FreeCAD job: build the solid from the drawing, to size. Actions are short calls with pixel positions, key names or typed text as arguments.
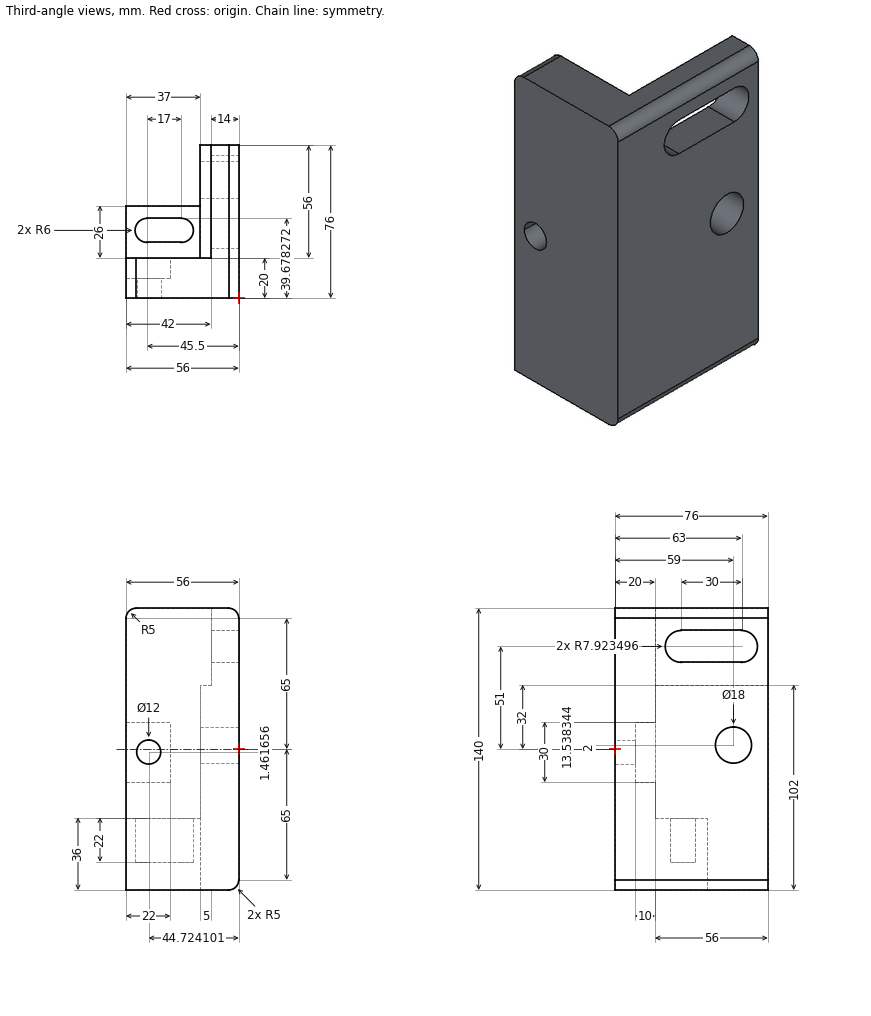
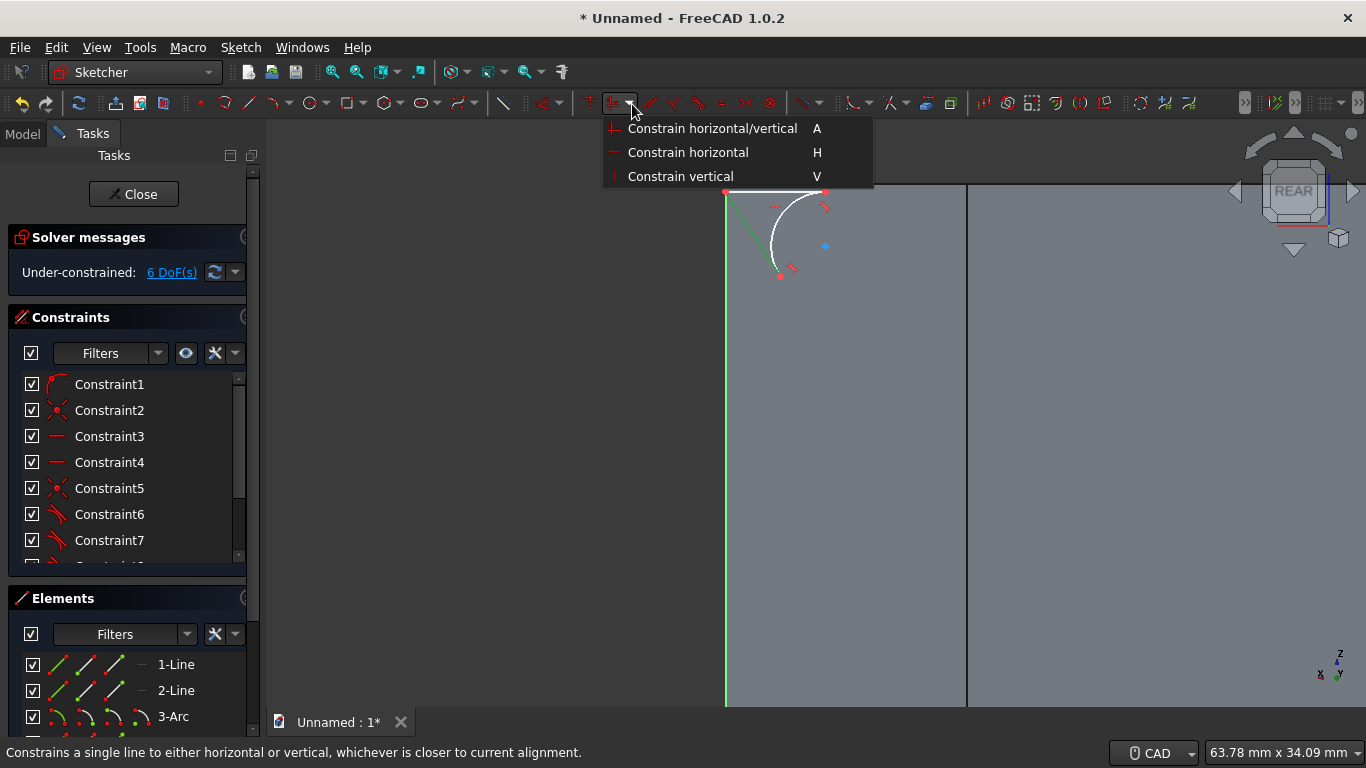
click(738, 176)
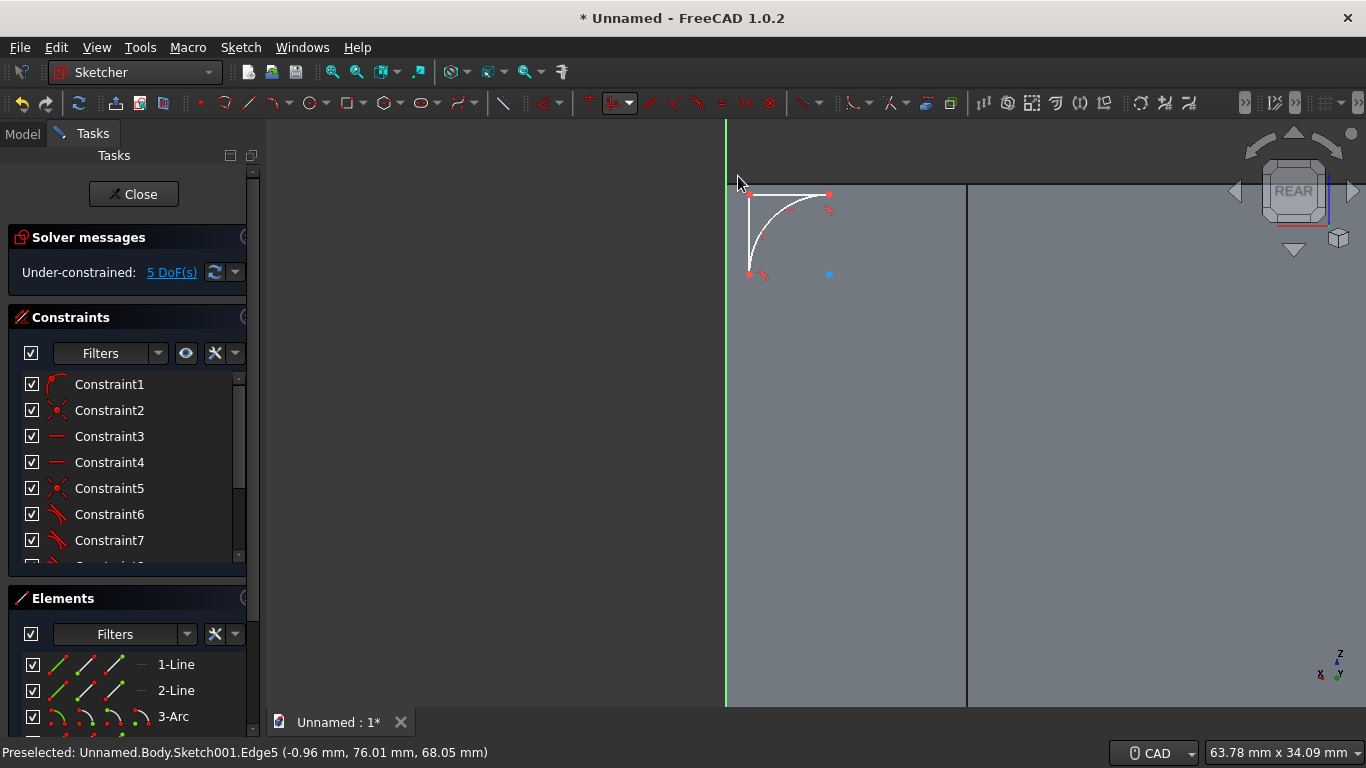
scroll(743, 219, down, 9)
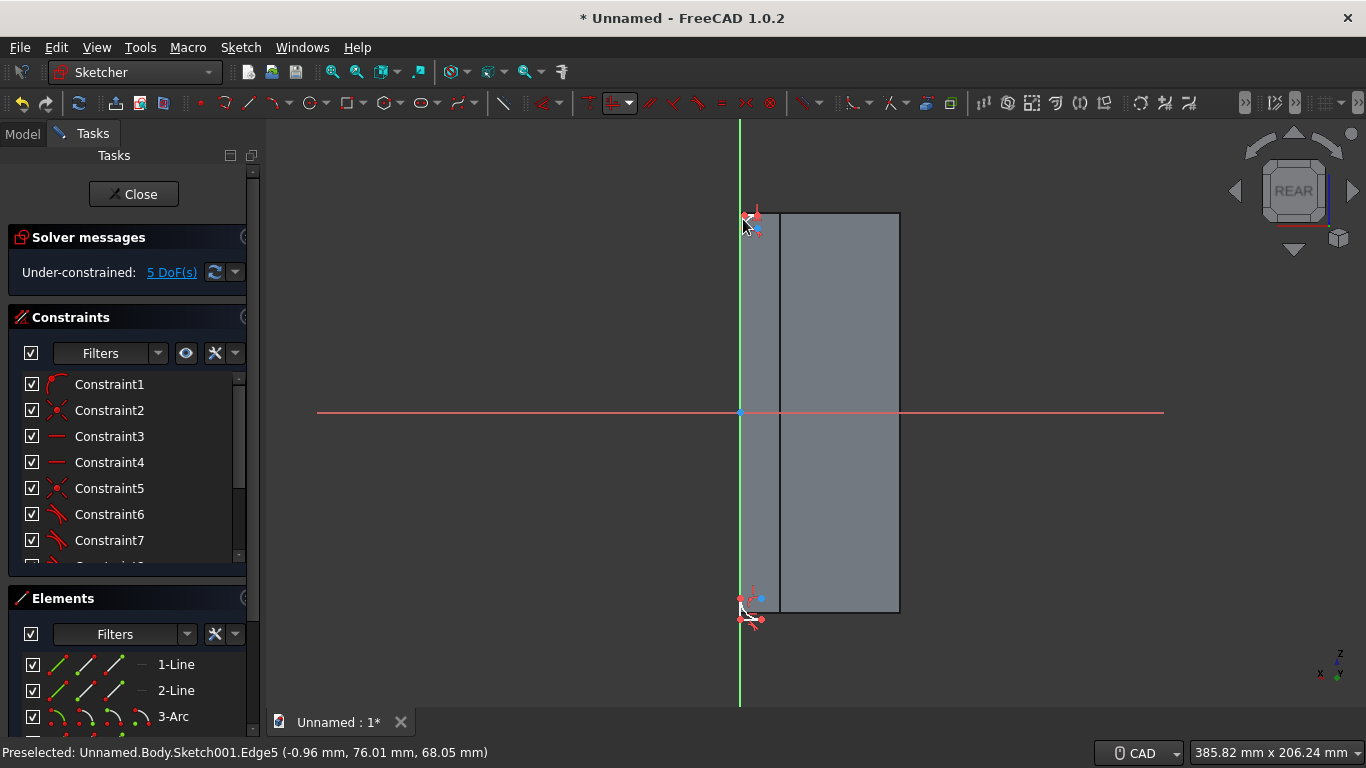
scroll(743, 608, up, 9)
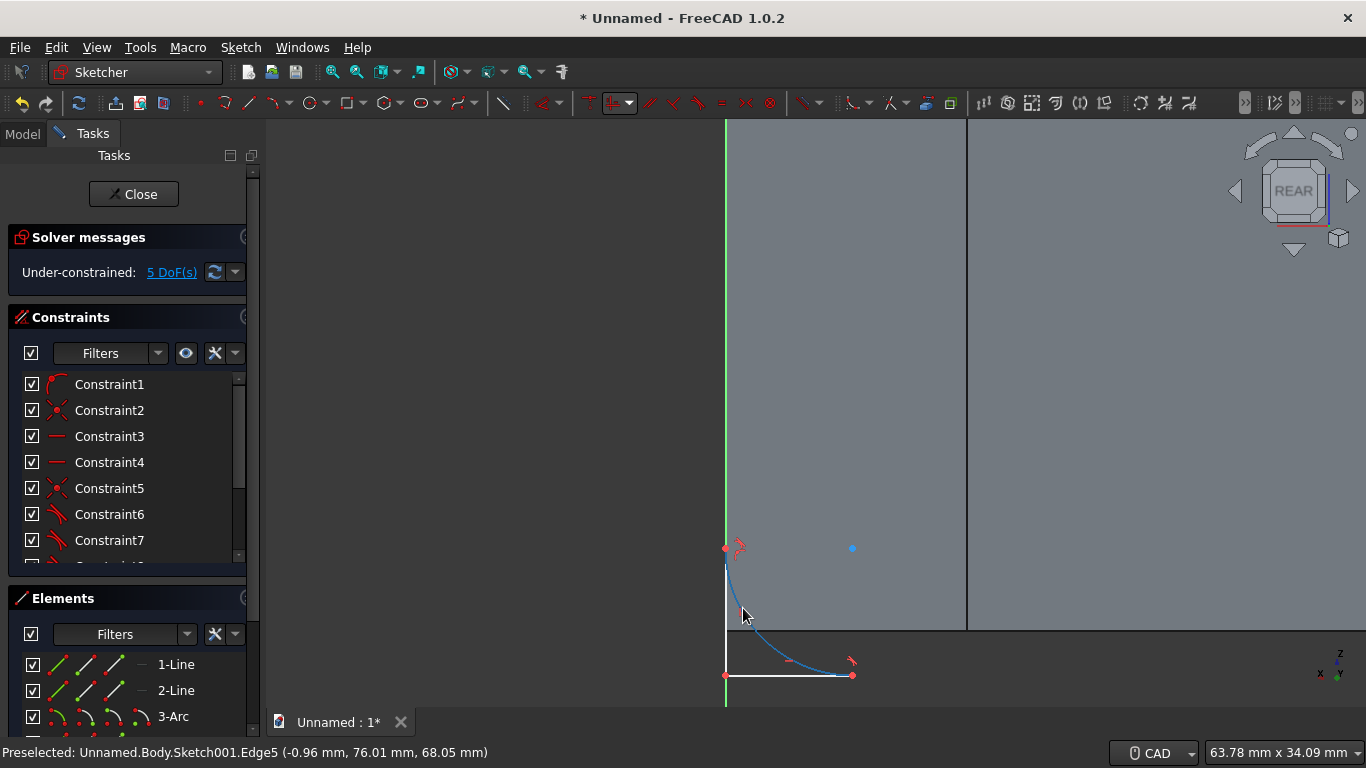
click(763, 638)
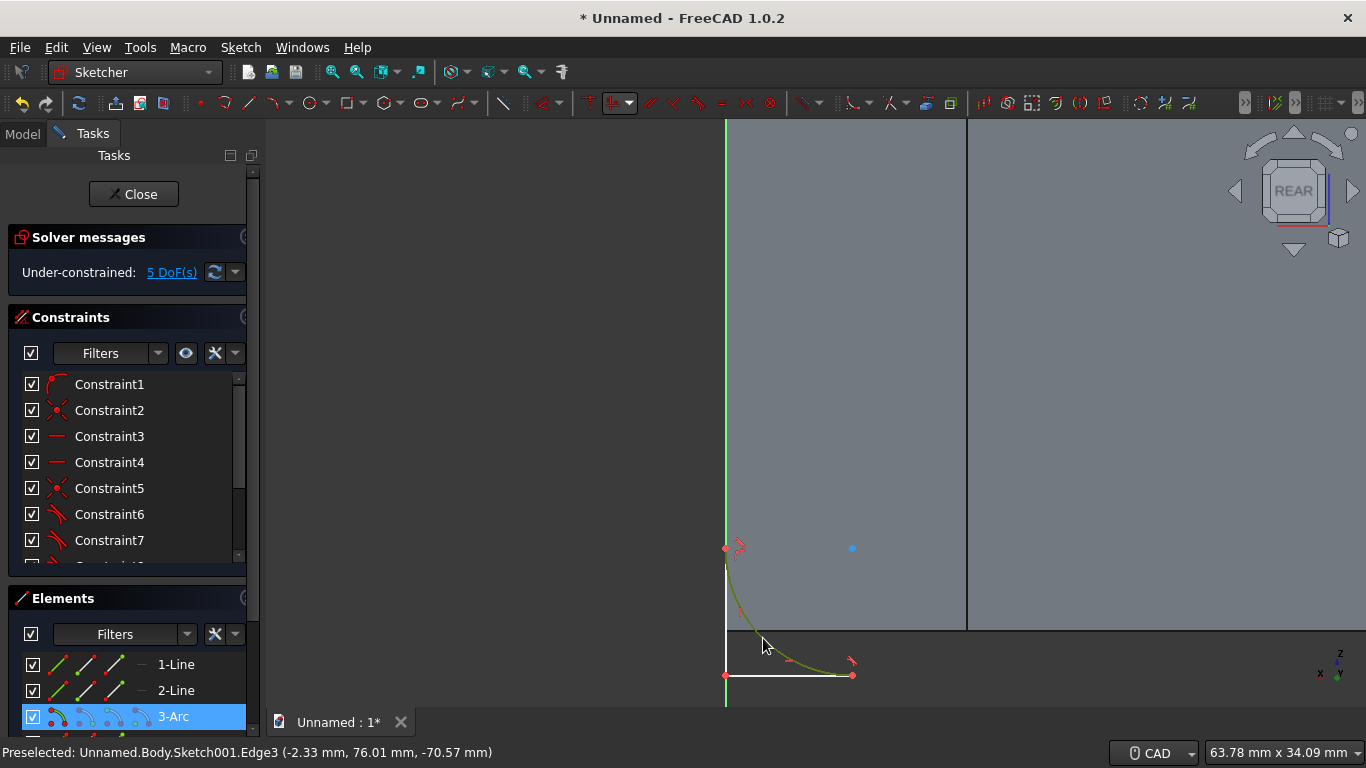
scroll(743, 609, down, 9)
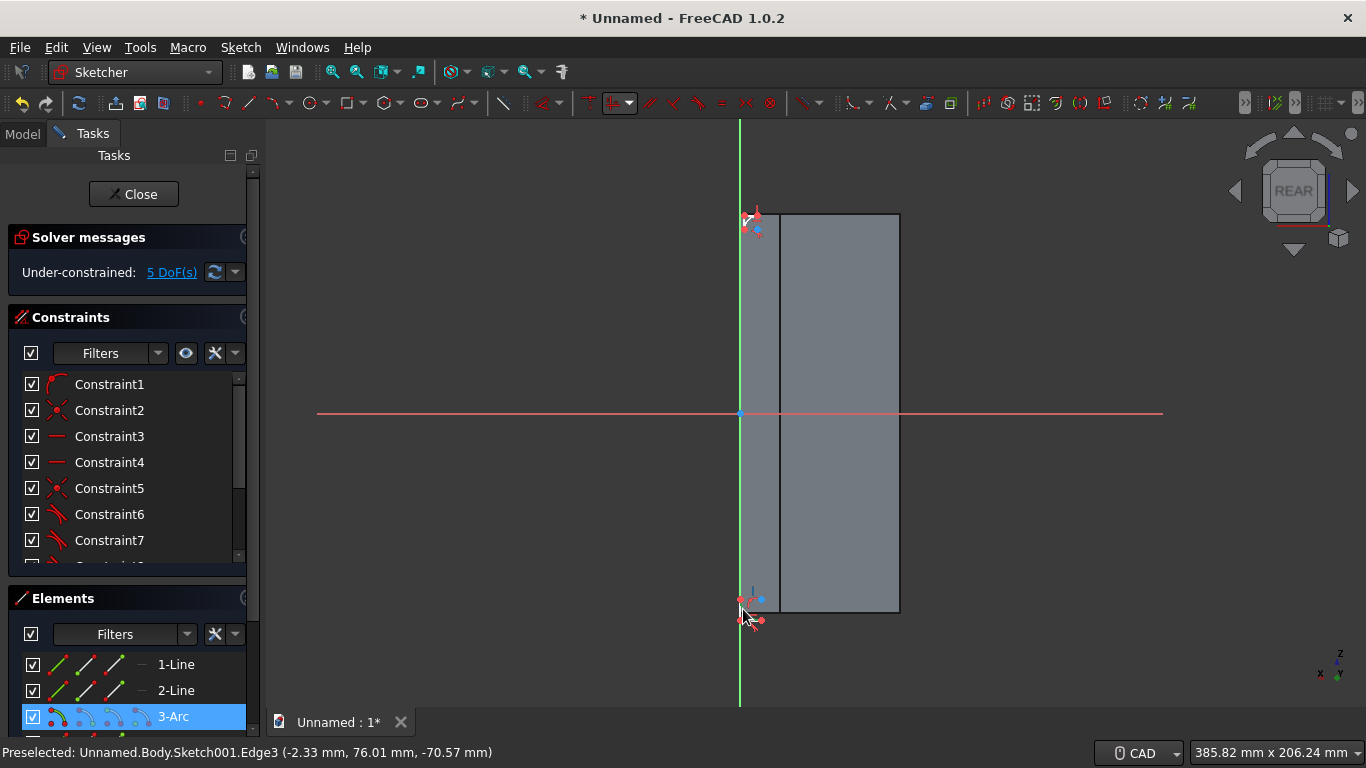
scroll(748, 220, up, 7)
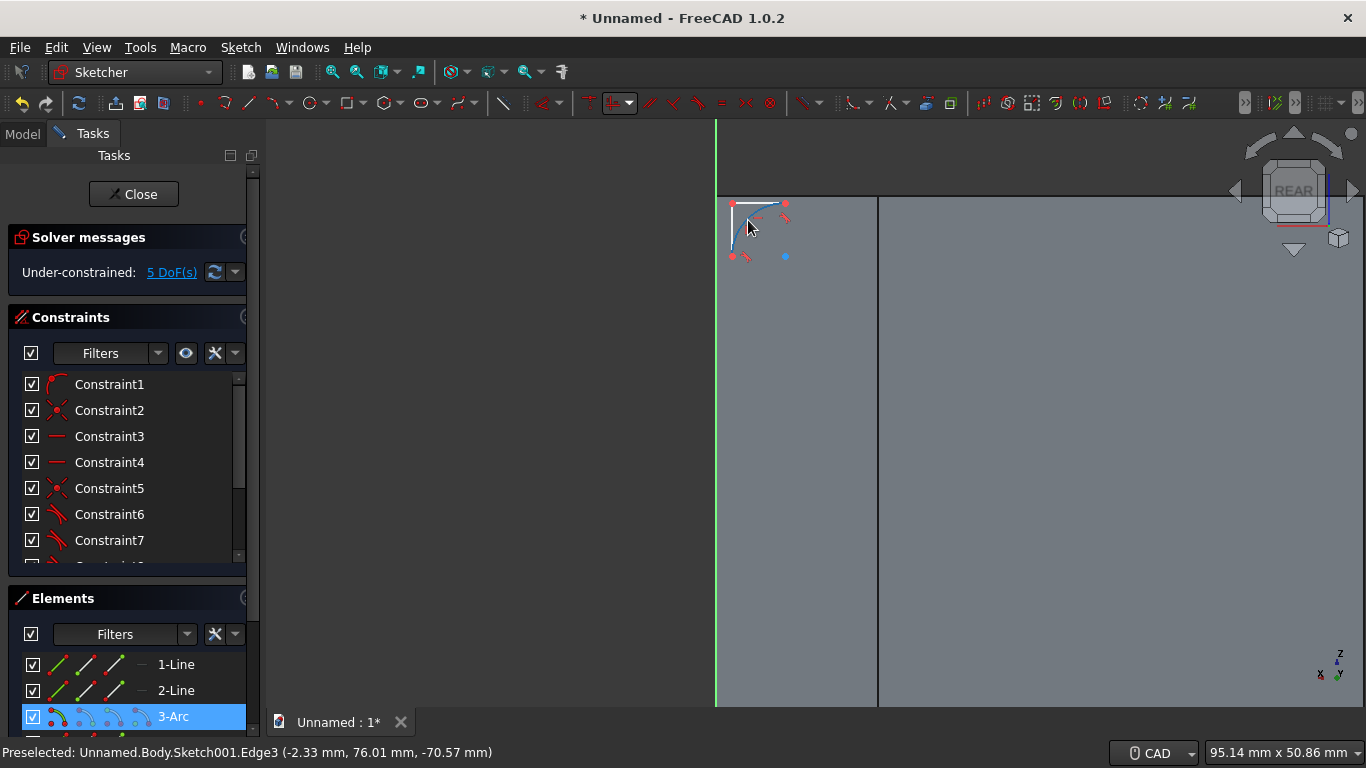
click(748, 219)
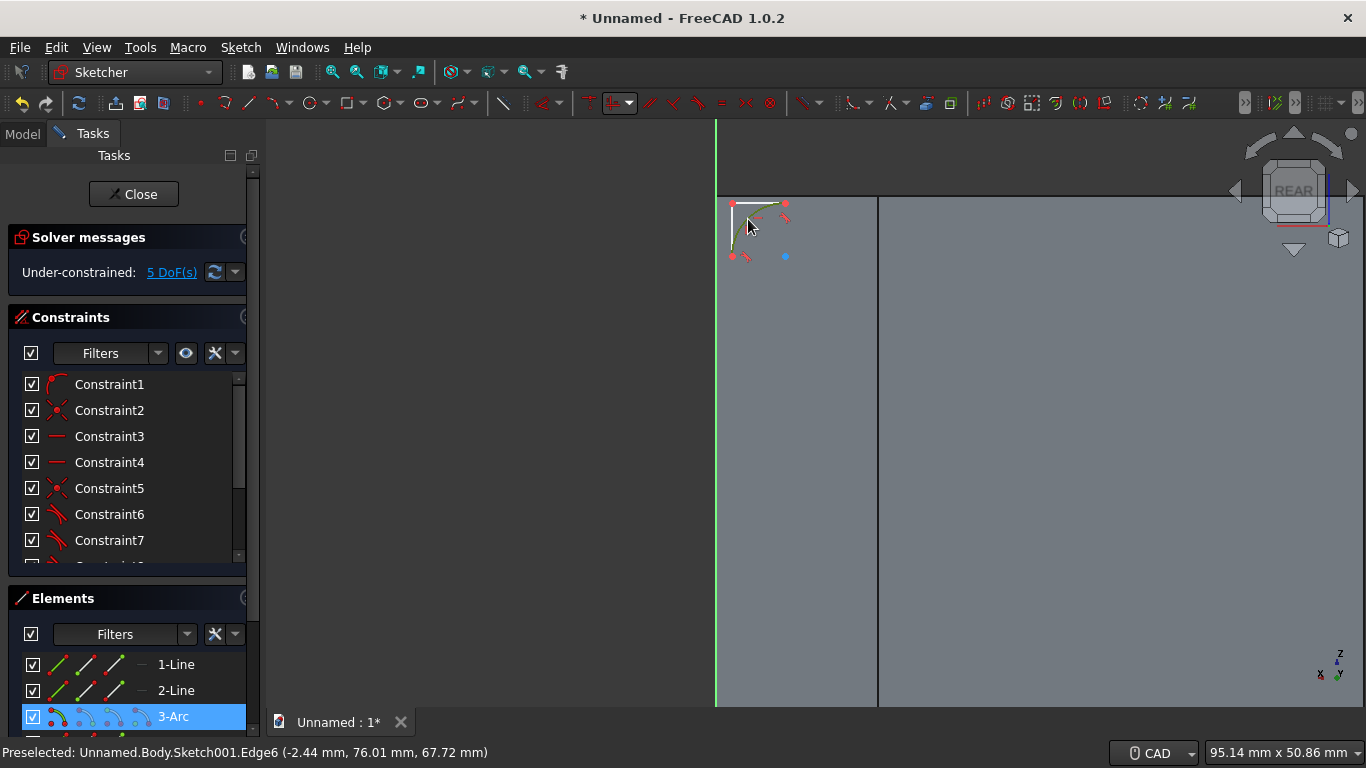
click(722, 104)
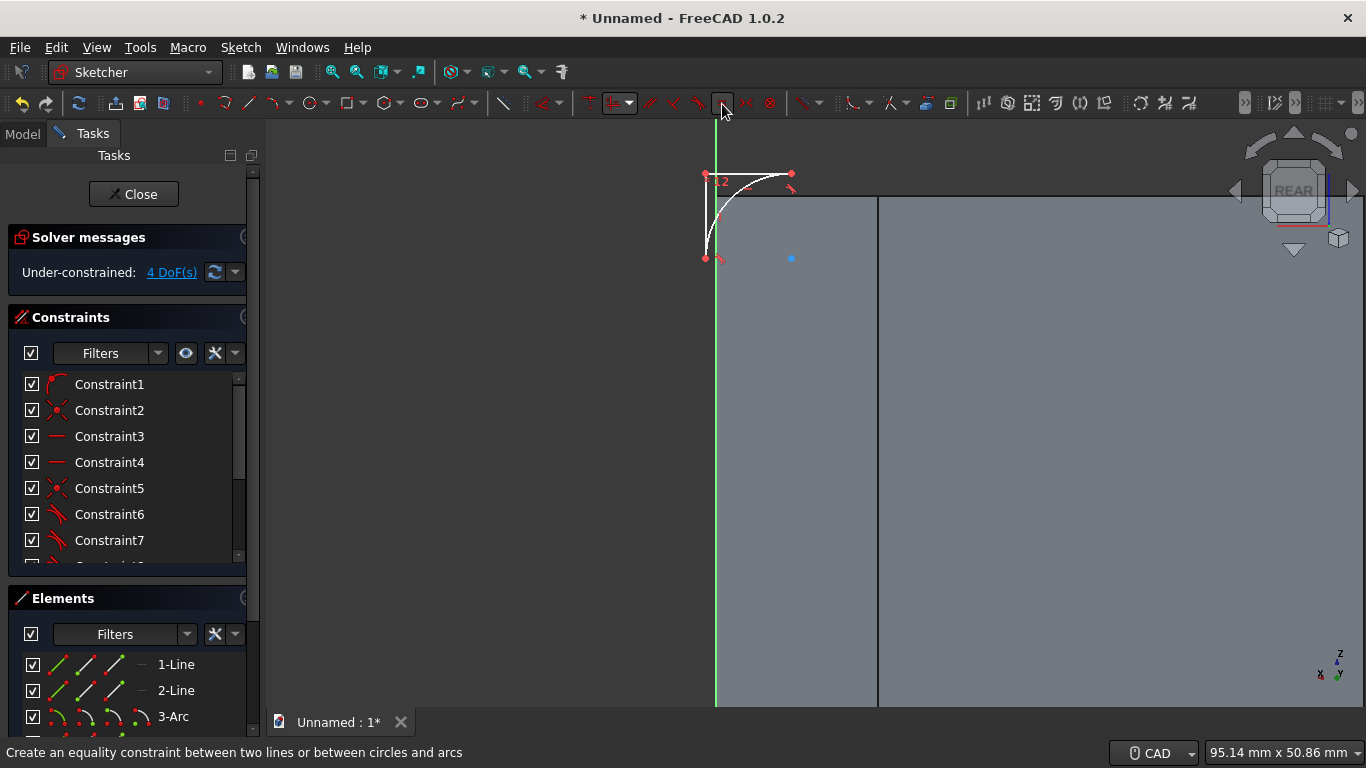
scroll(748, 219, down, 7)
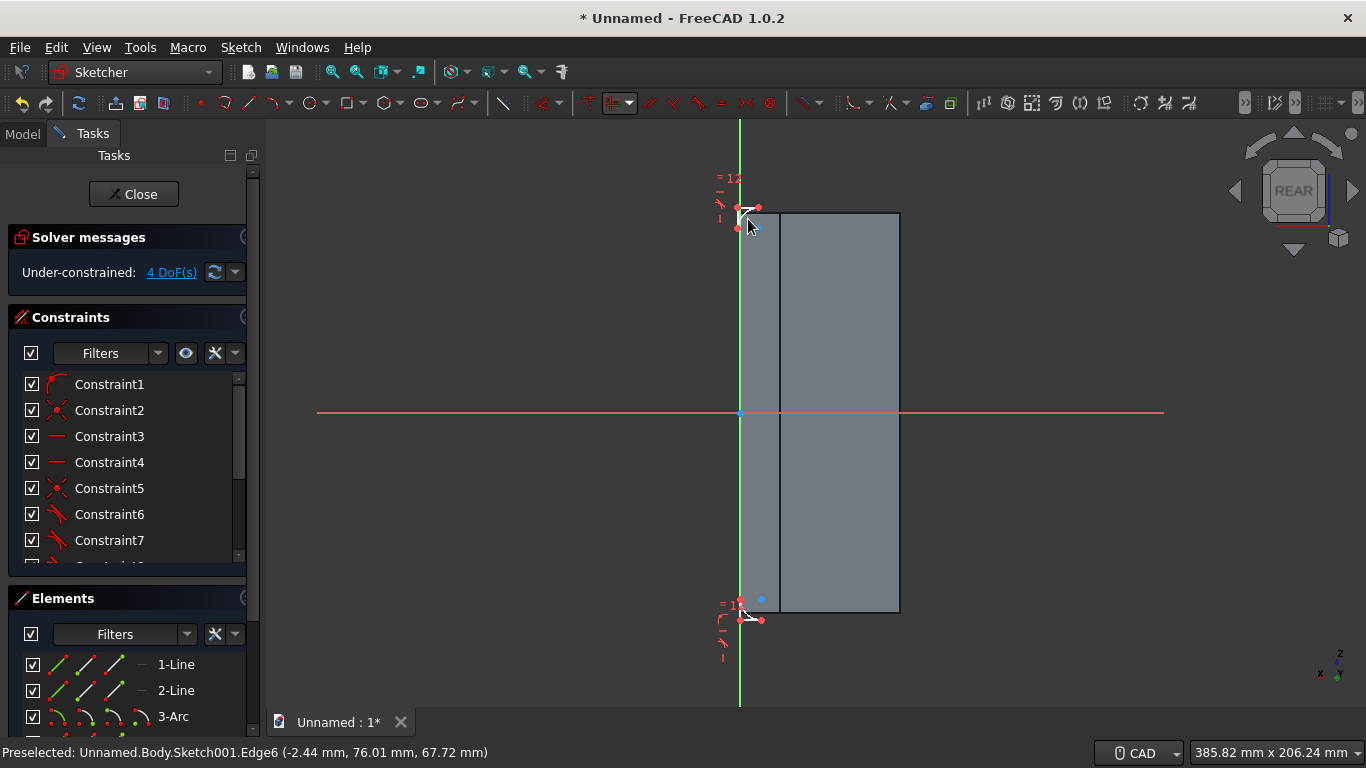
click(761, 599)